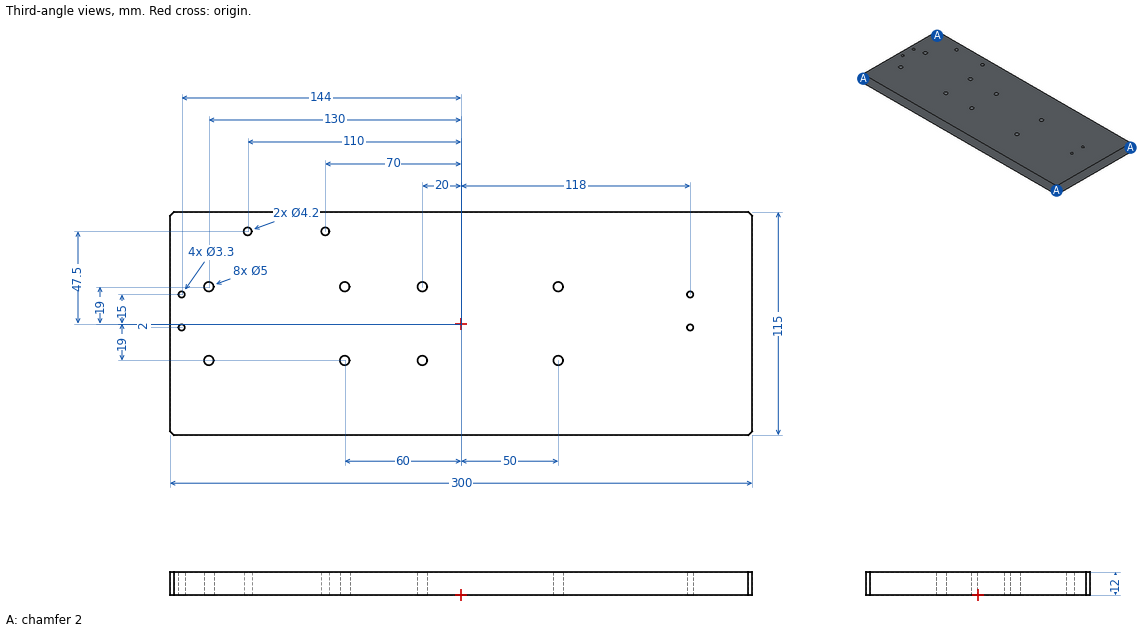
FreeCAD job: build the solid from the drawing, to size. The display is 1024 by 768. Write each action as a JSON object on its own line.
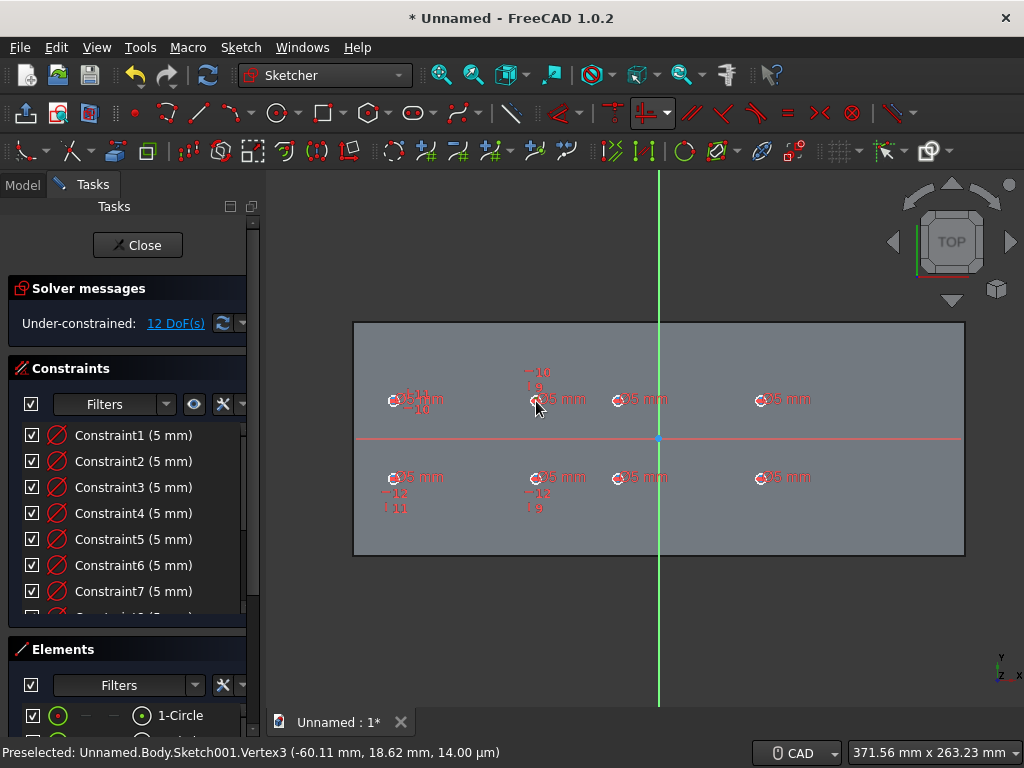
{"action": "left_click", "coordinate": [618, 401]}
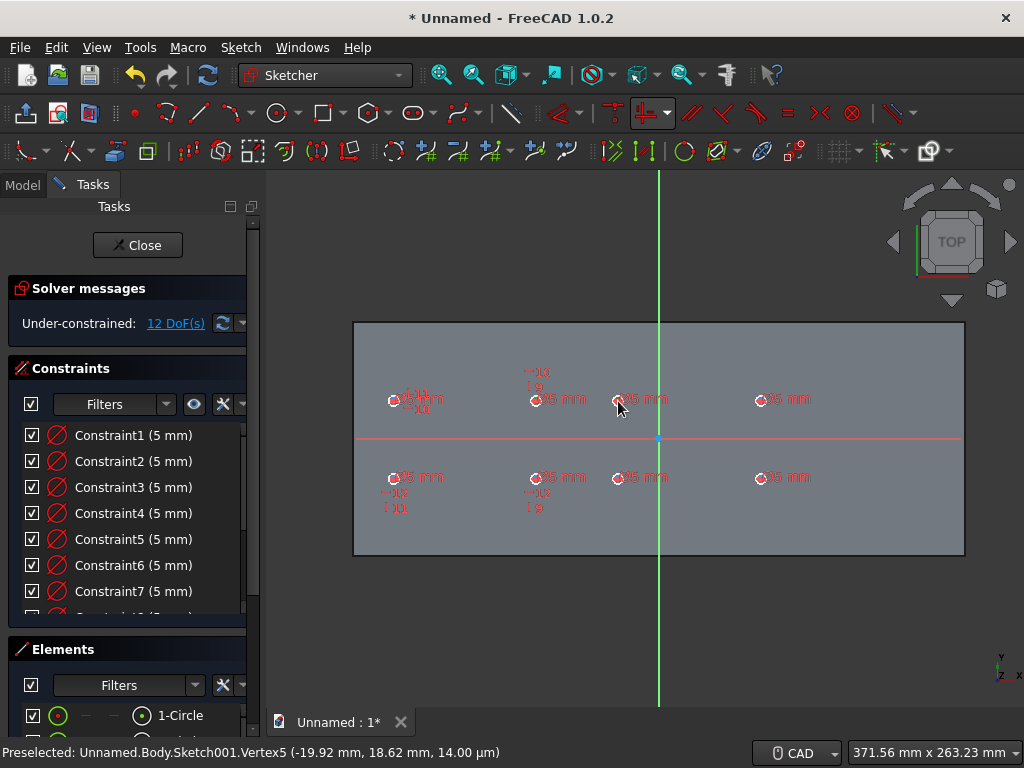
{"action": "left_click", "coordinate": [670, 114]}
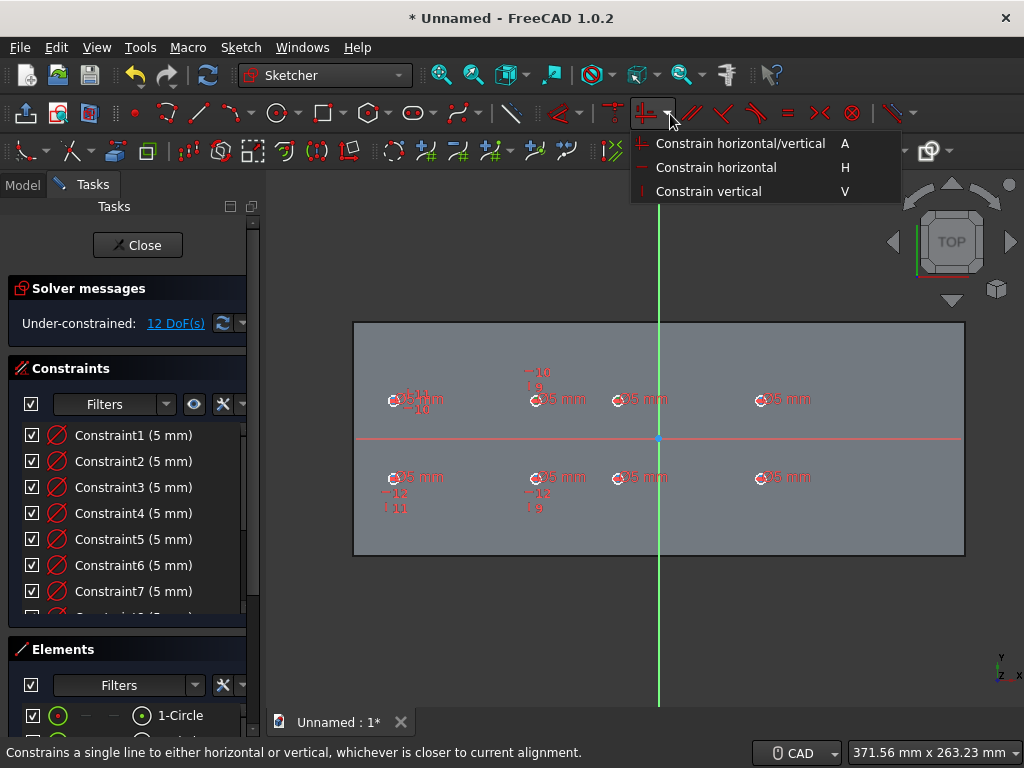
{"action": "left_click", "coordinate": [766, 167]}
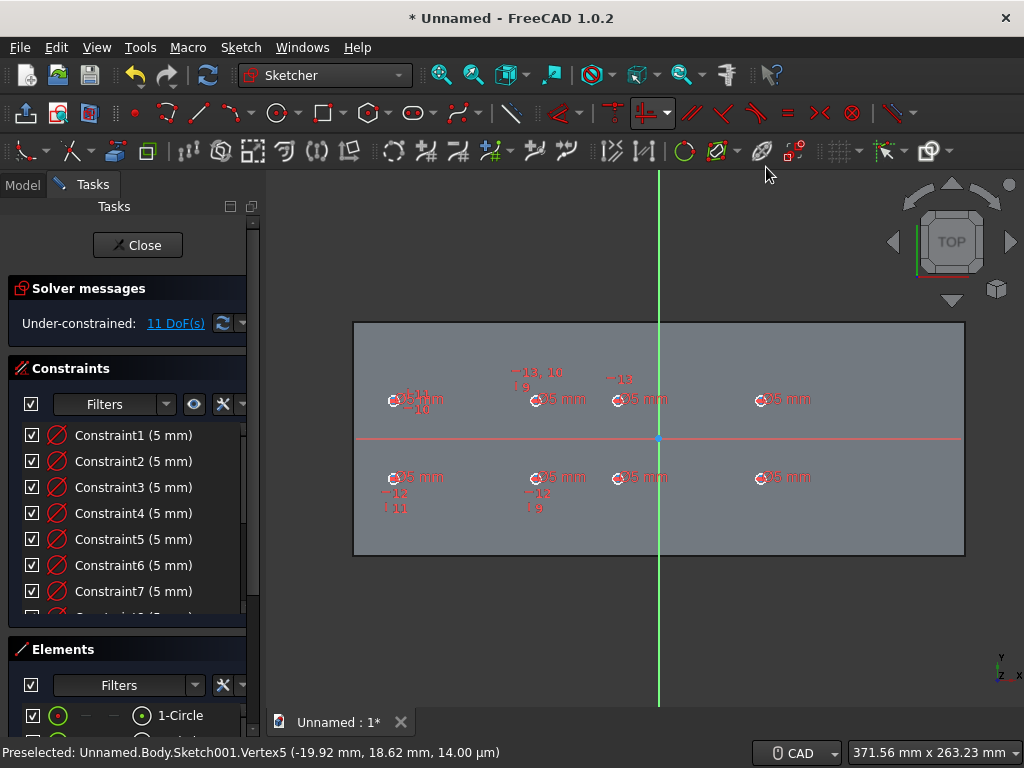
{"action": "left_click", "coordinate": [536, 479]}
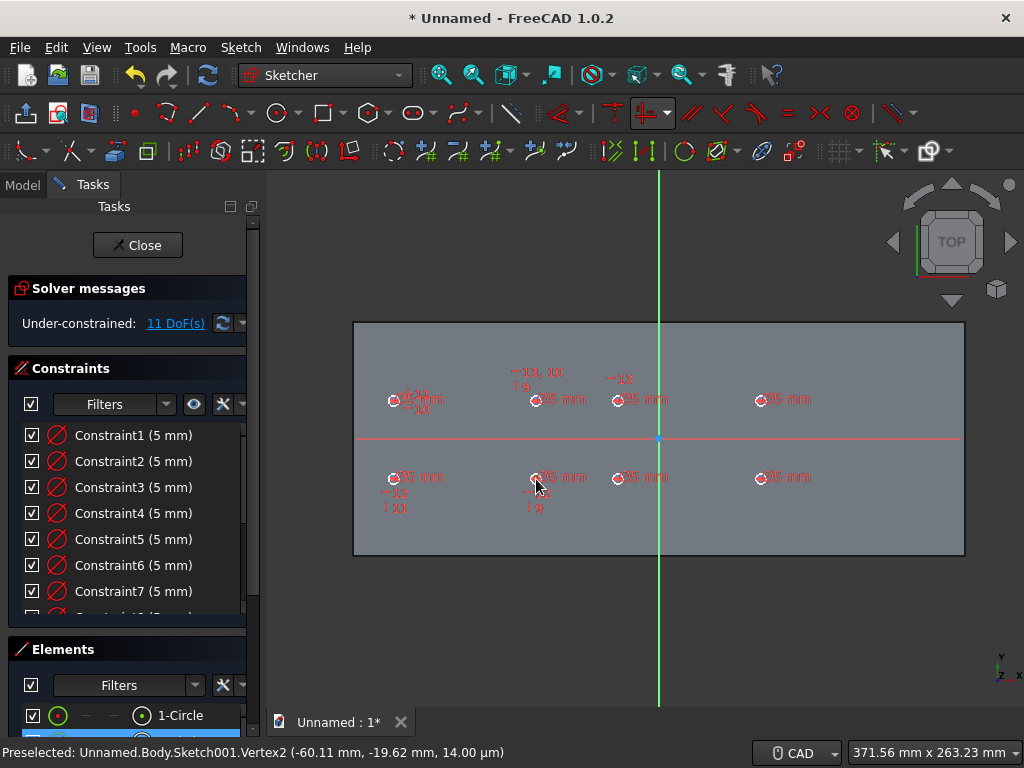
{"action": "left_click", "coordinate": [761, 479]}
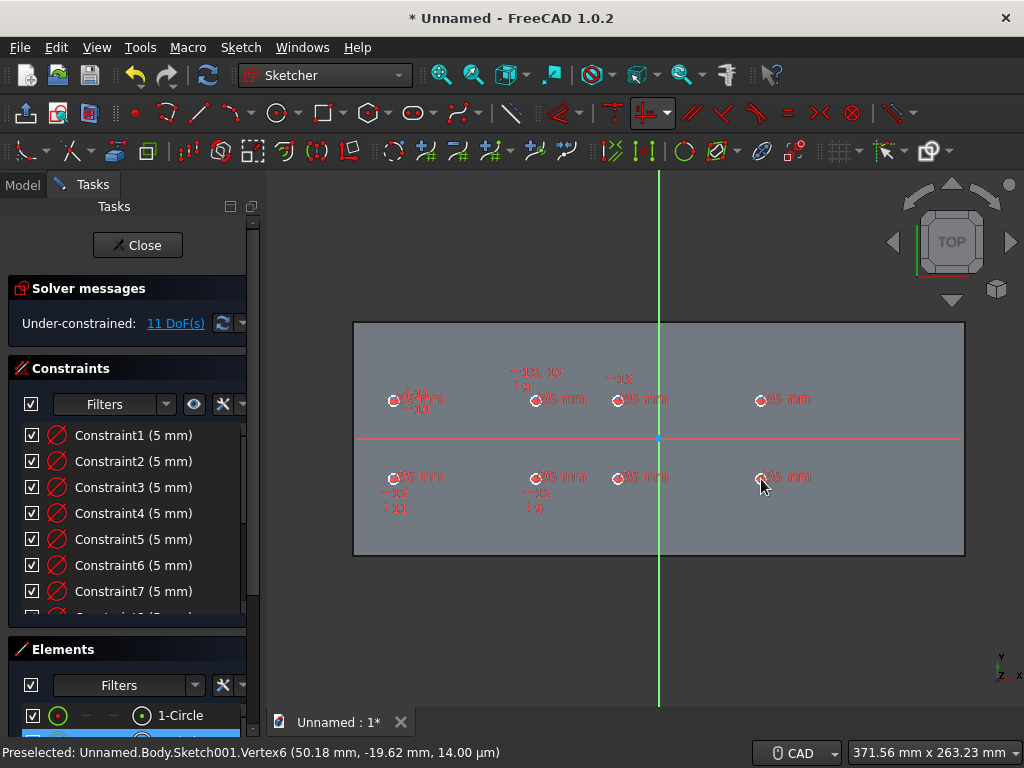
{"action": "left_click", "coordinate": [670, 114]}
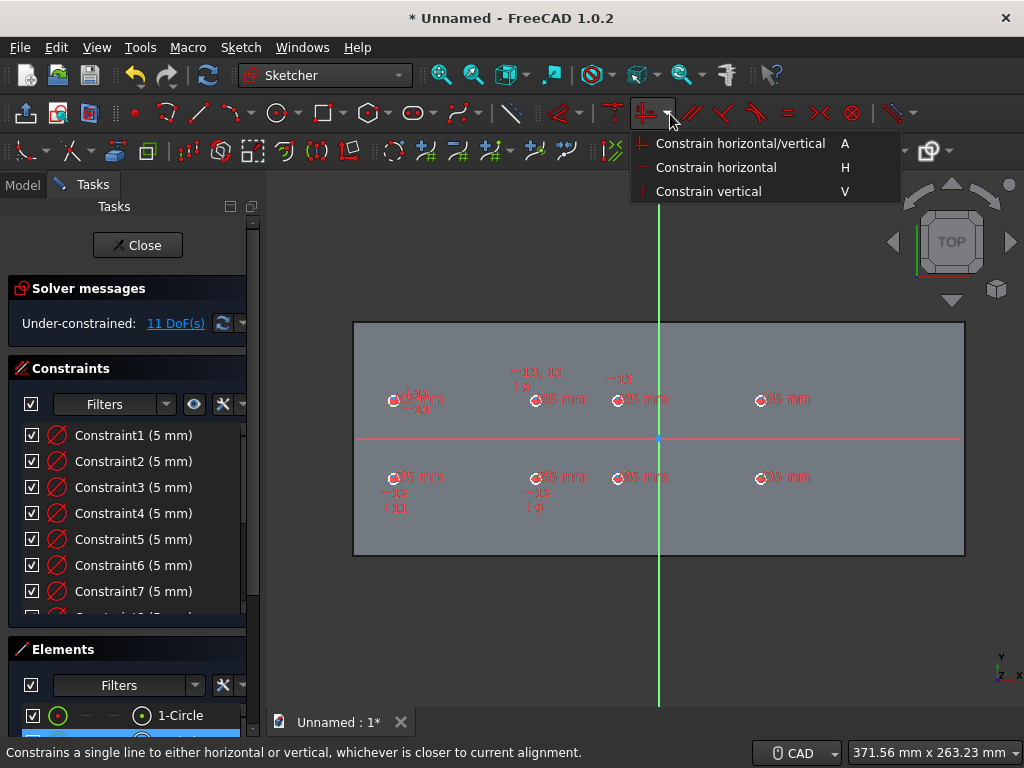
{"action": "left_click", "coordinate": [766, 167]}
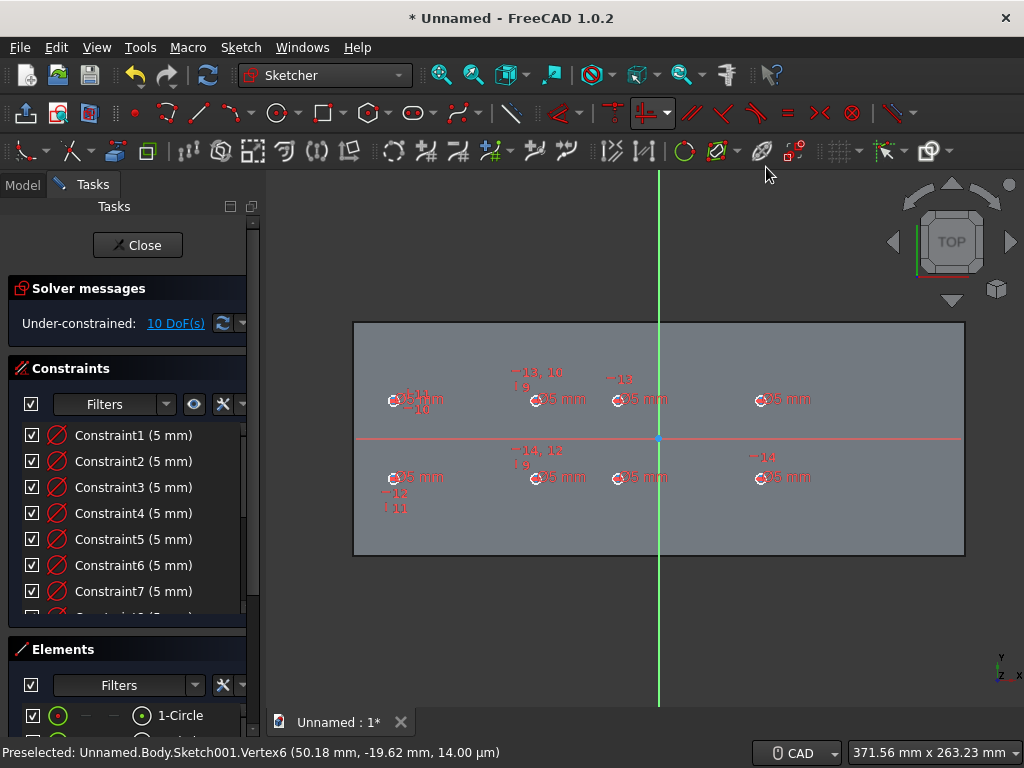
{"action": "left_click", "coordinate": [761, 479]}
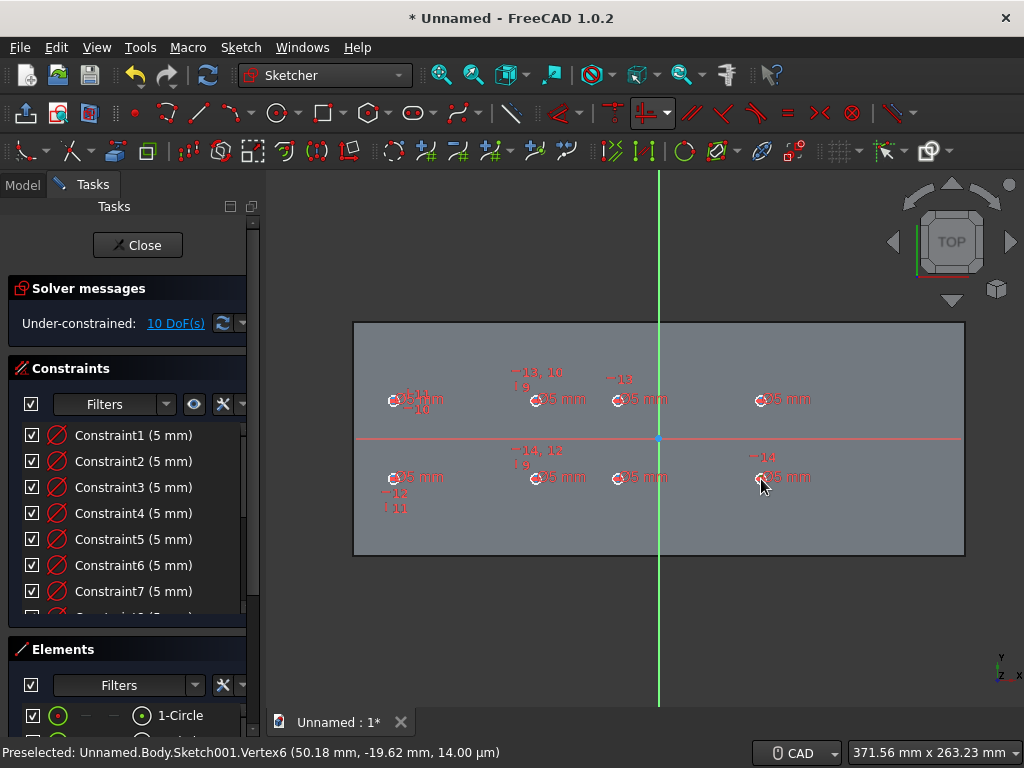
{"action": "left_click", "coordinate": [761, 401]}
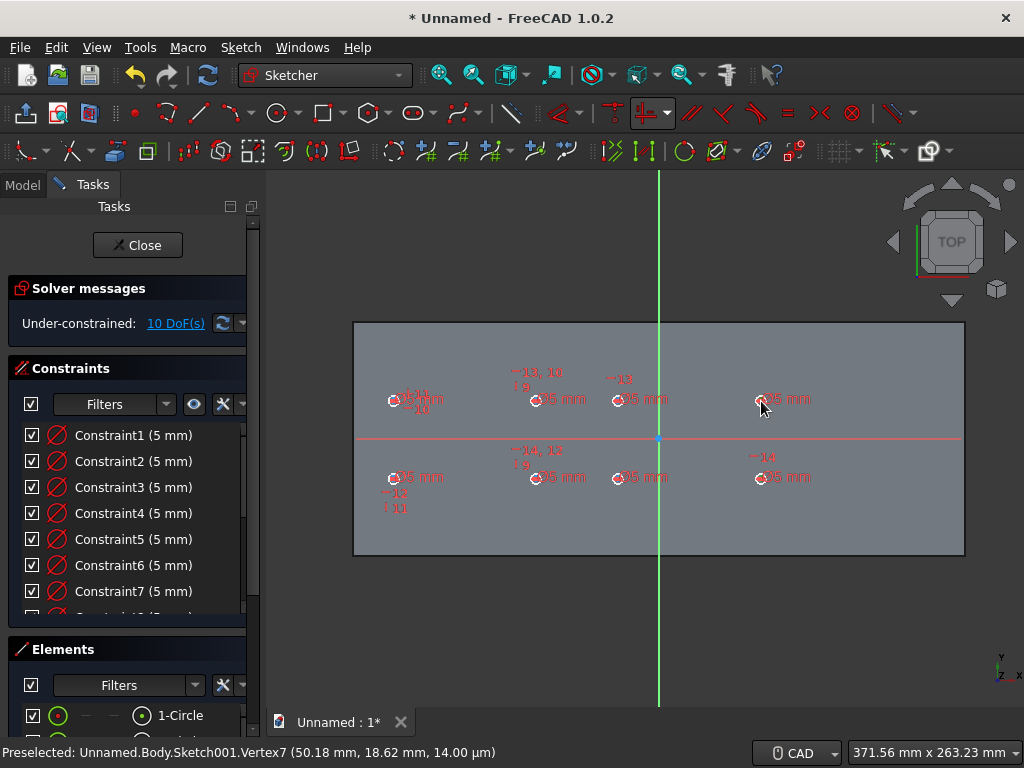
{"action": "key", "text": "v"}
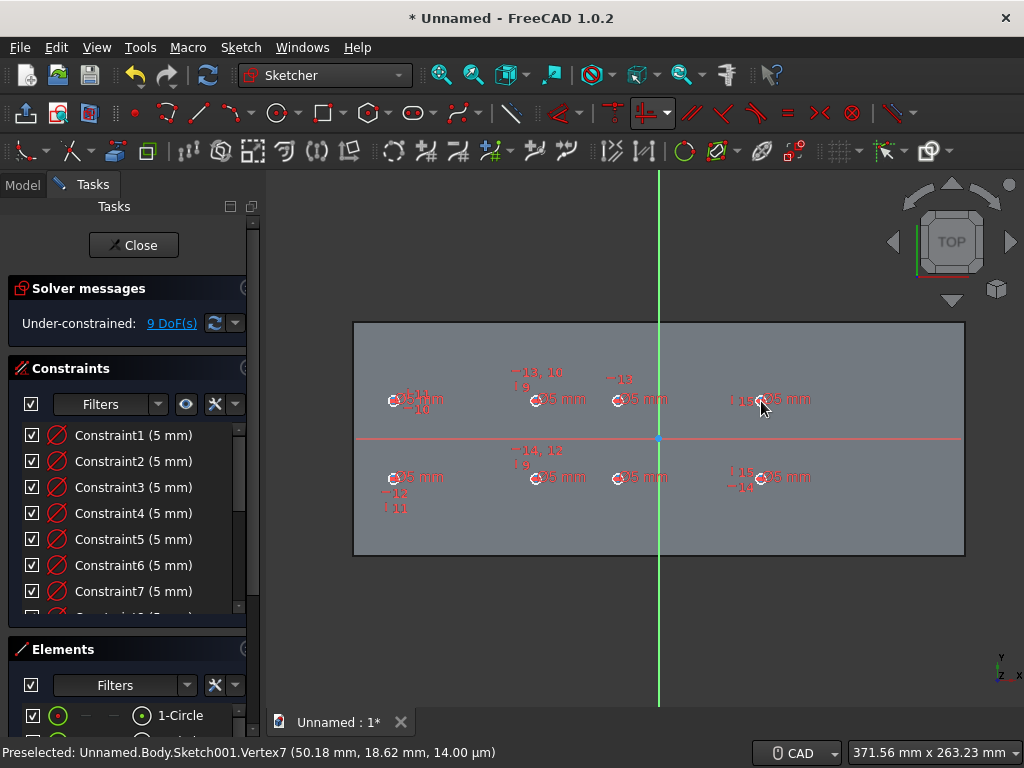
{"action": "left_click", "coordinate": [618, 401]}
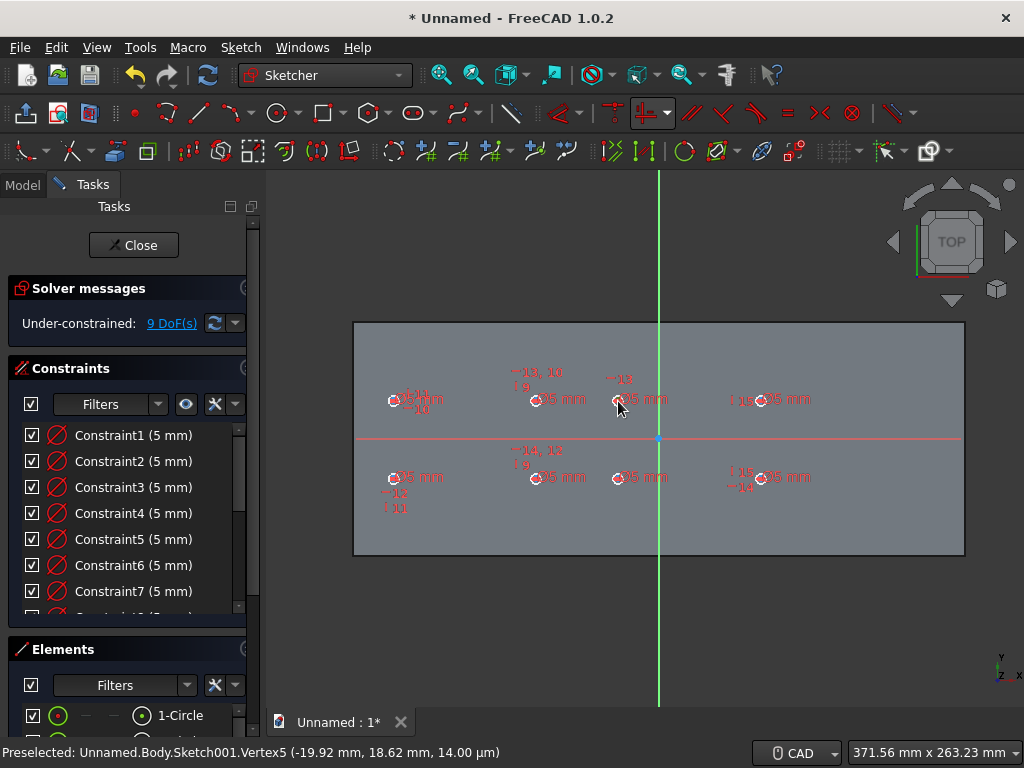
{"action": "left_click", "coordinate": [761, 401]}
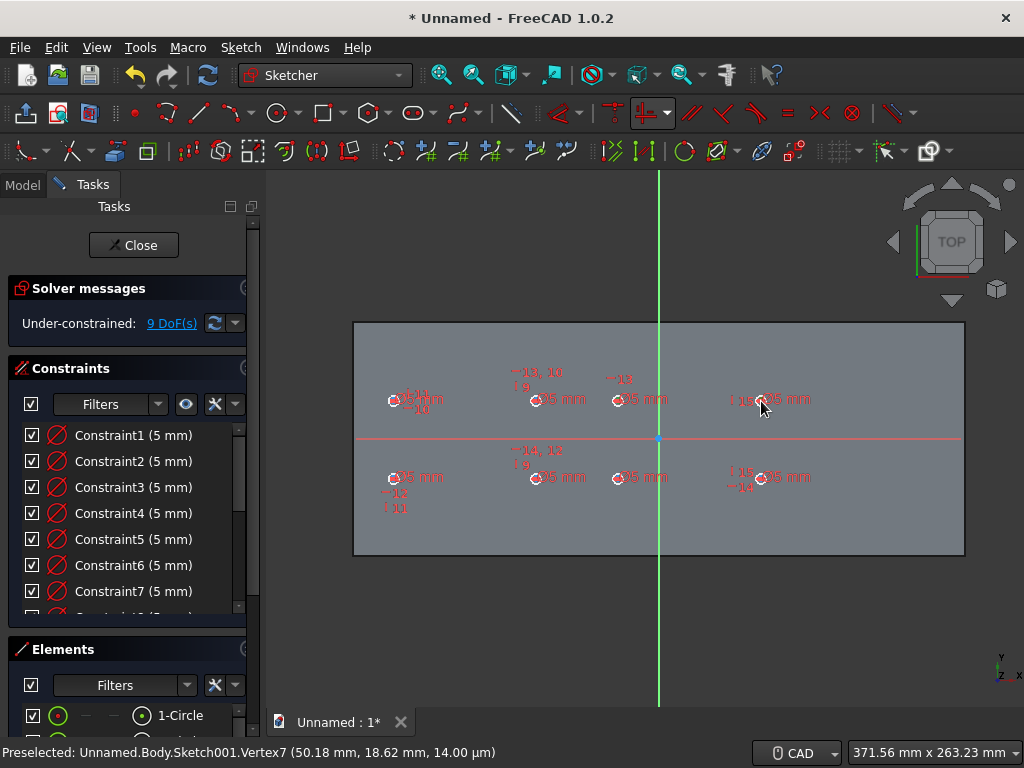
{"action": "key", "text": "h"}